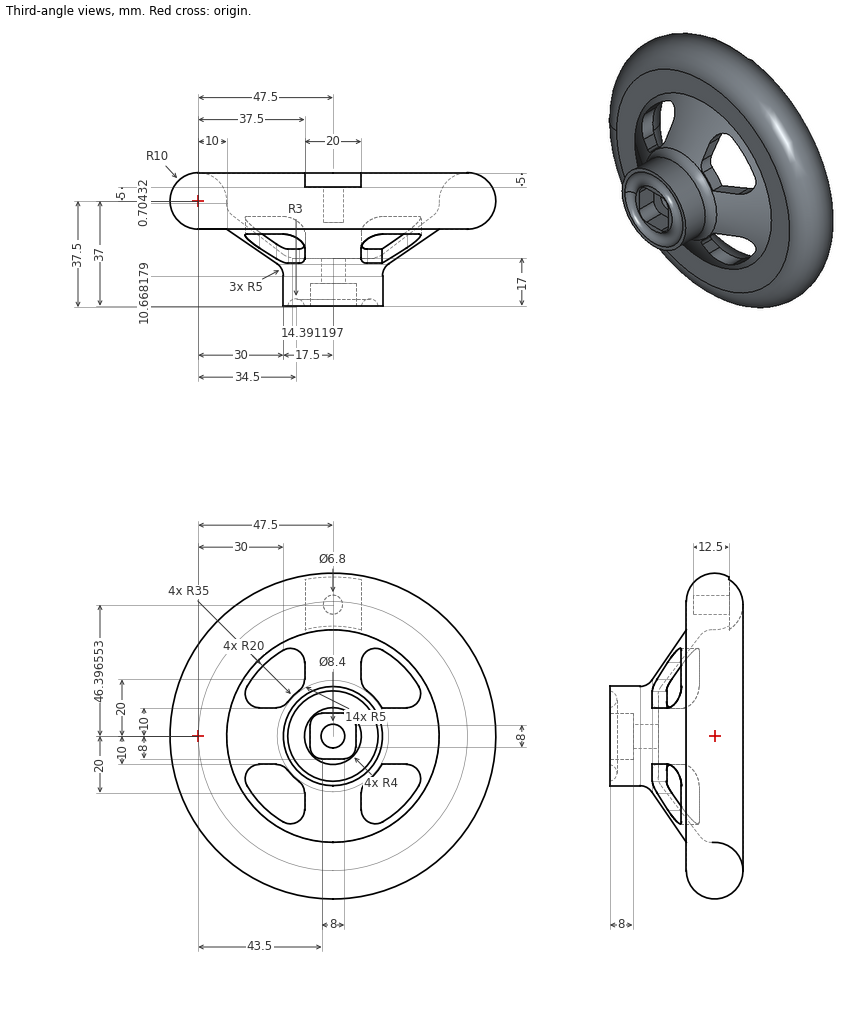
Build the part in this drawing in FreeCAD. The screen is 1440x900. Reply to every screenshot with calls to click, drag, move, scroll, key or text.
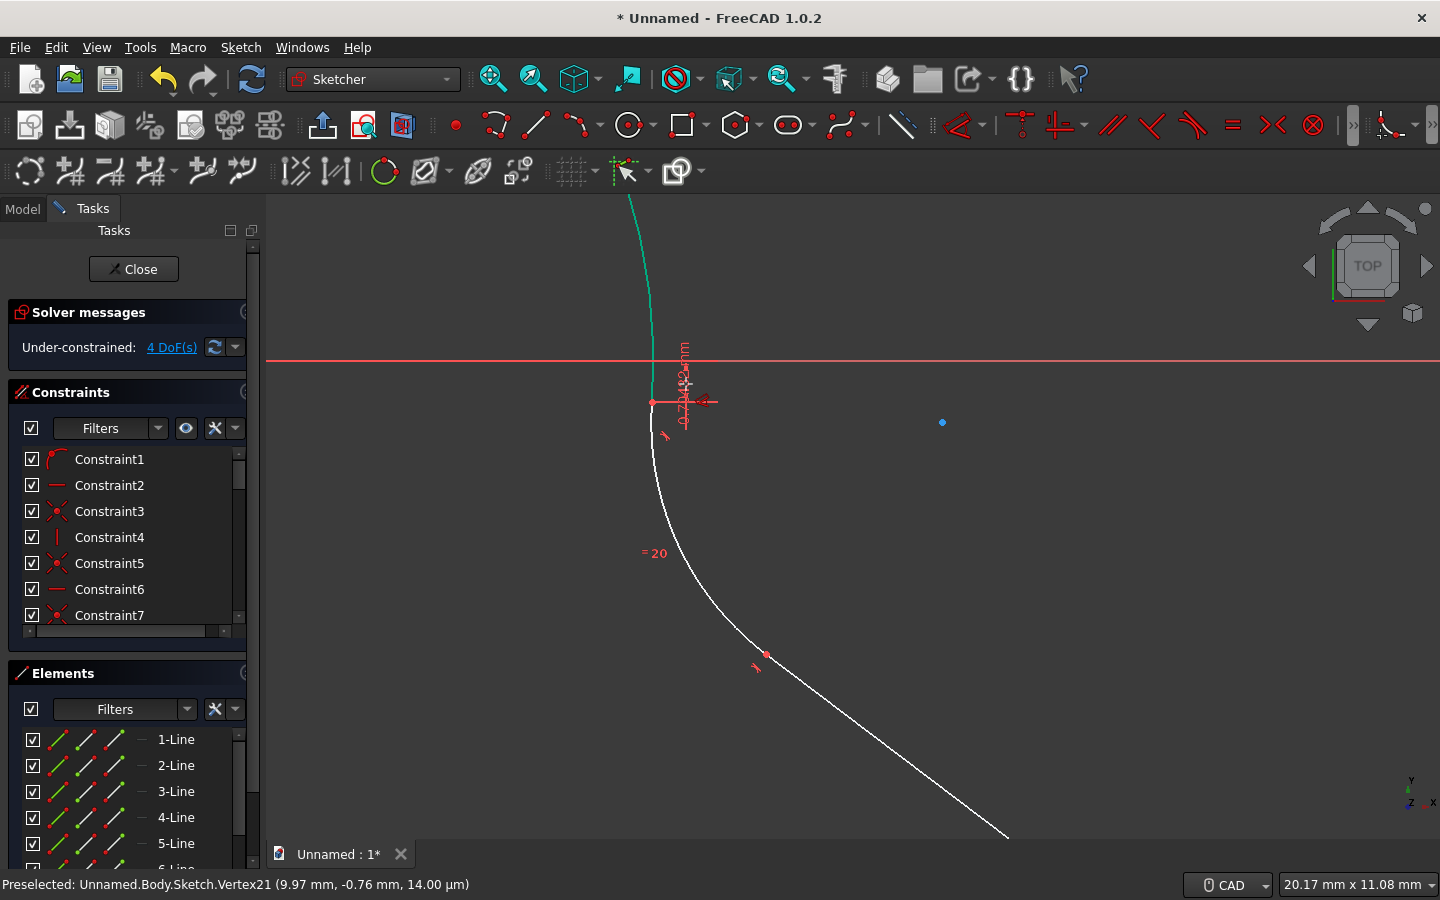
scroll(726, 492, down, 11)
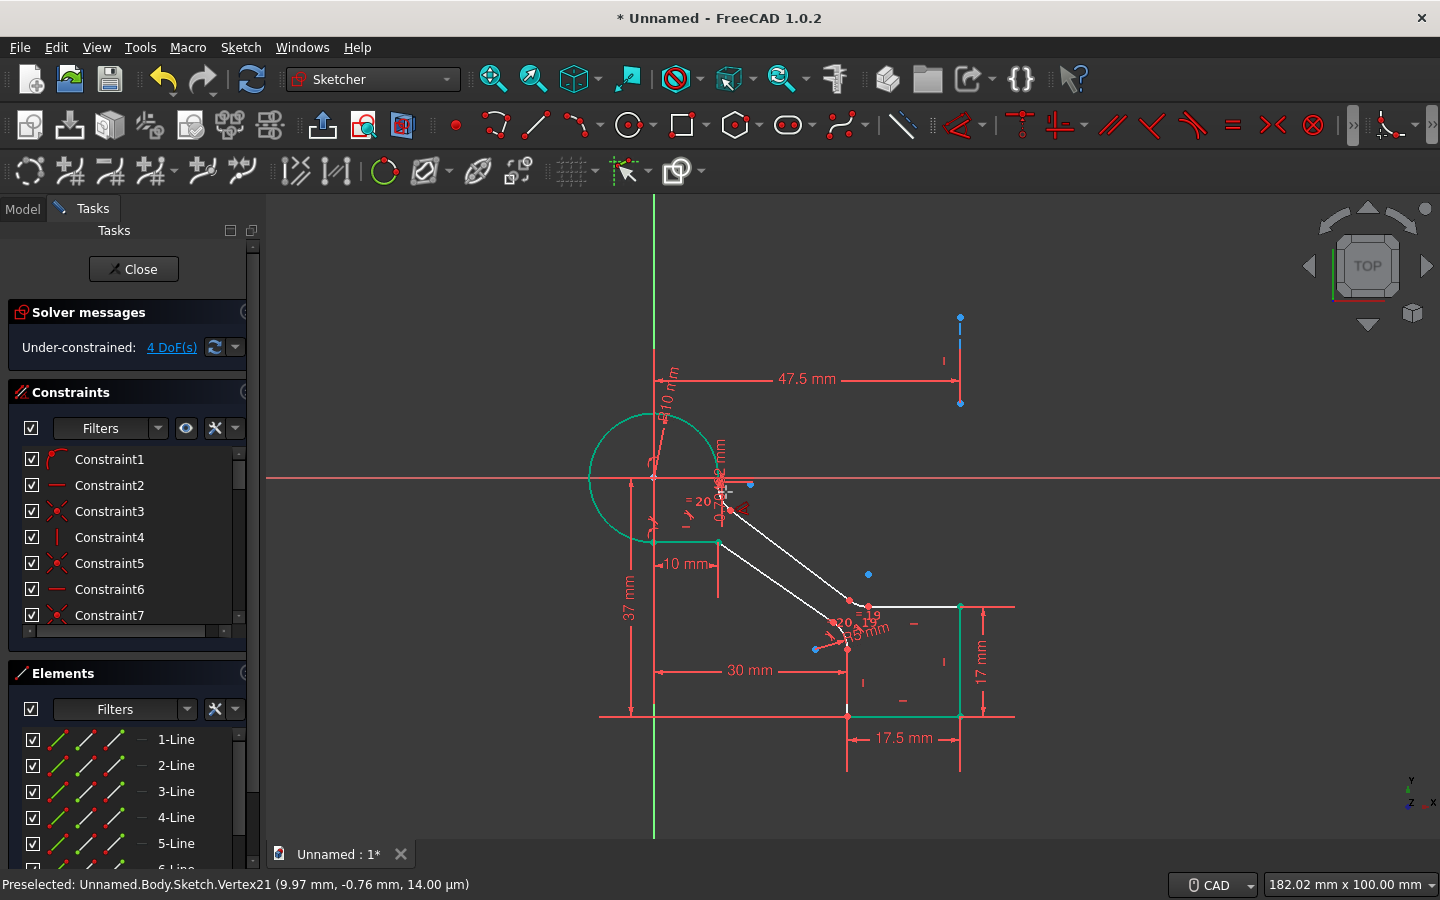
click(847, 669)
click(881, 683)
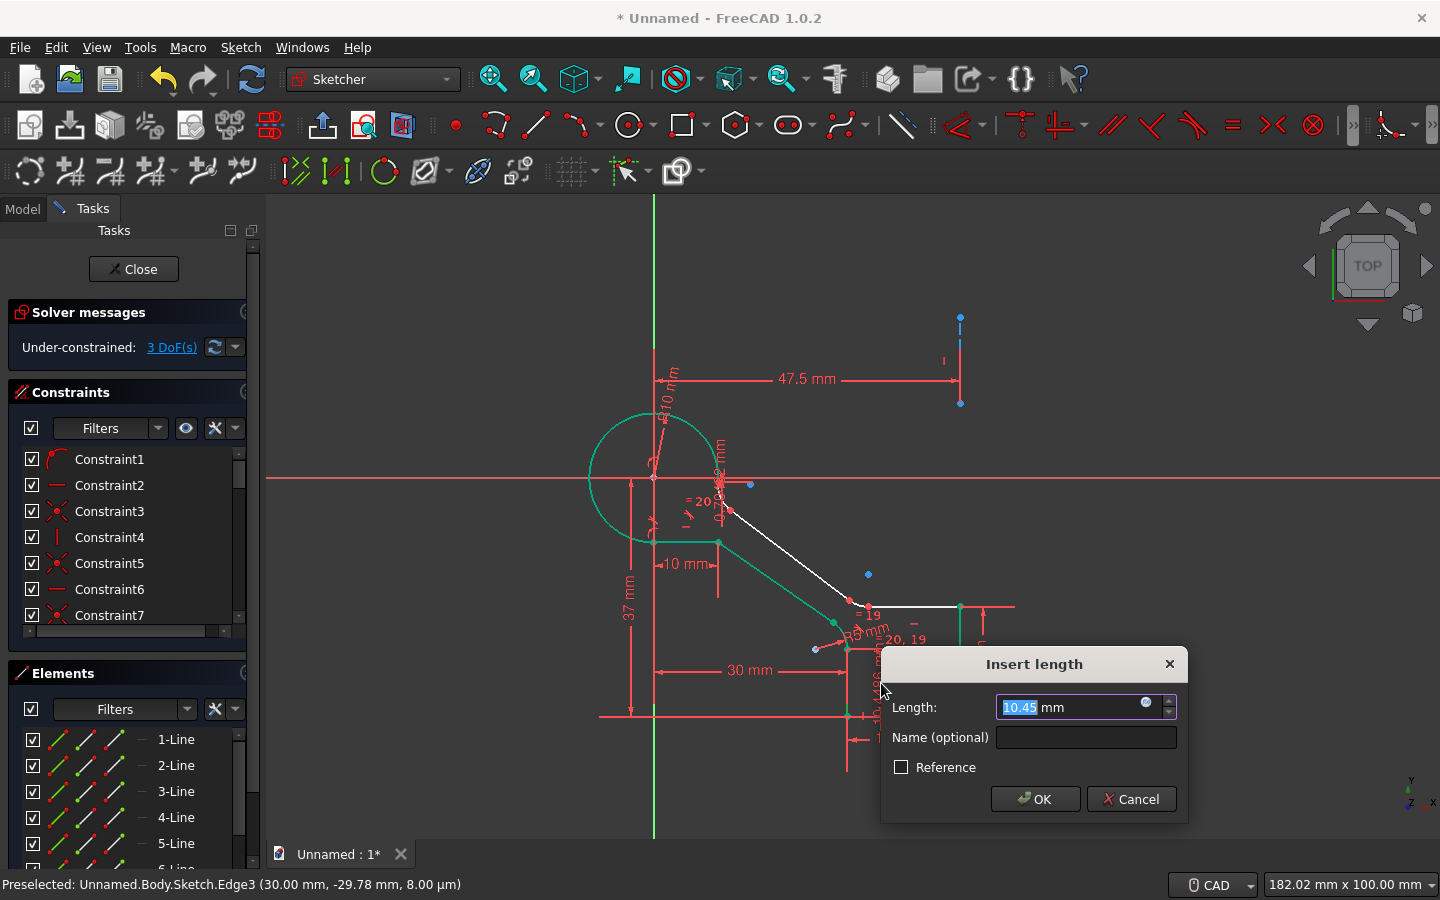
text(10.668179)
key(Return)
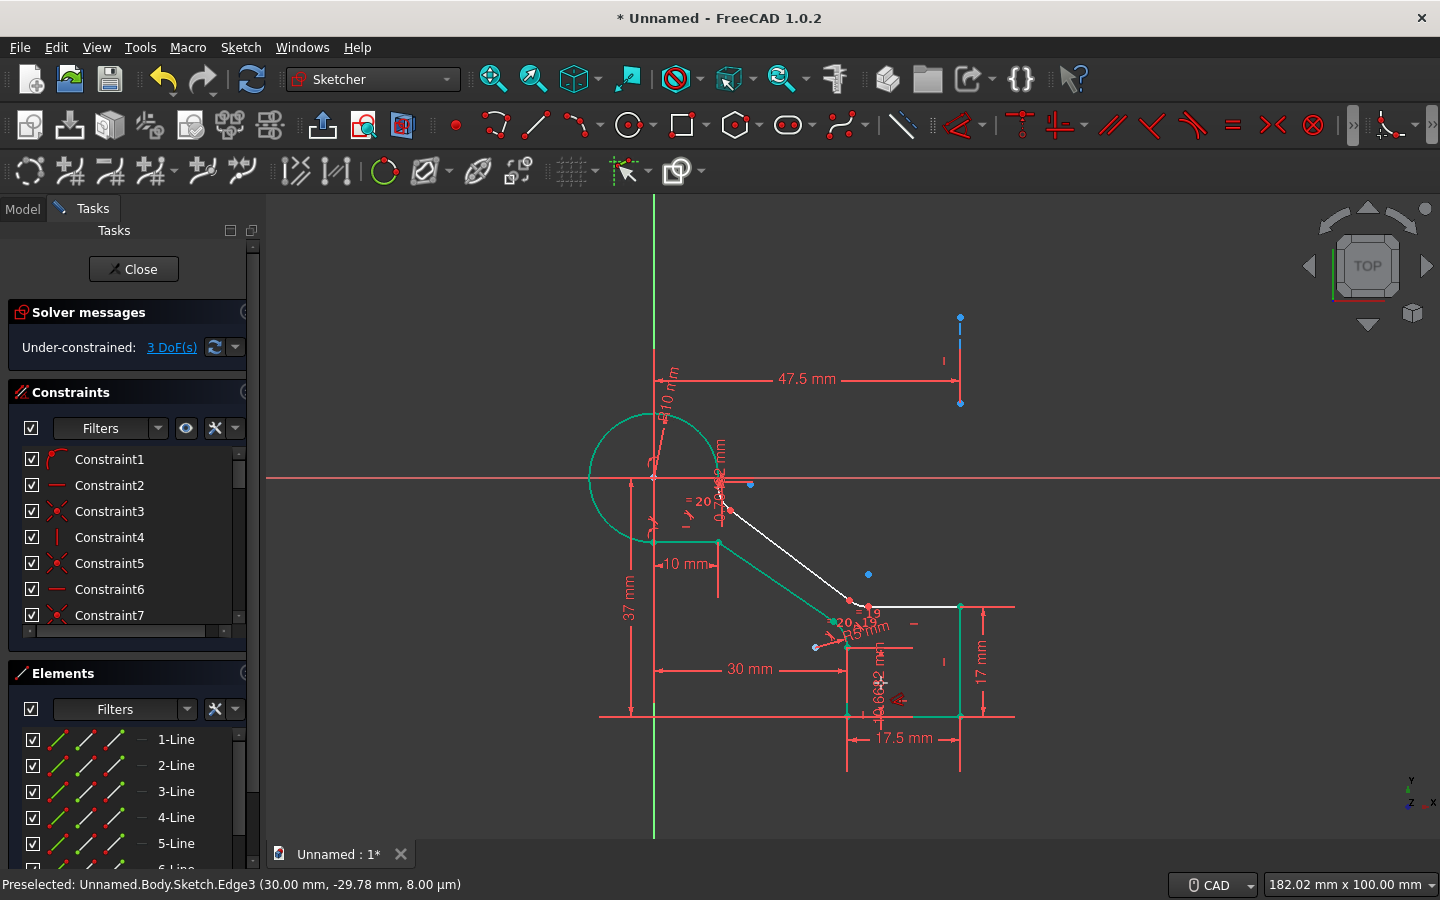
click(933, 607)
click(915, 573)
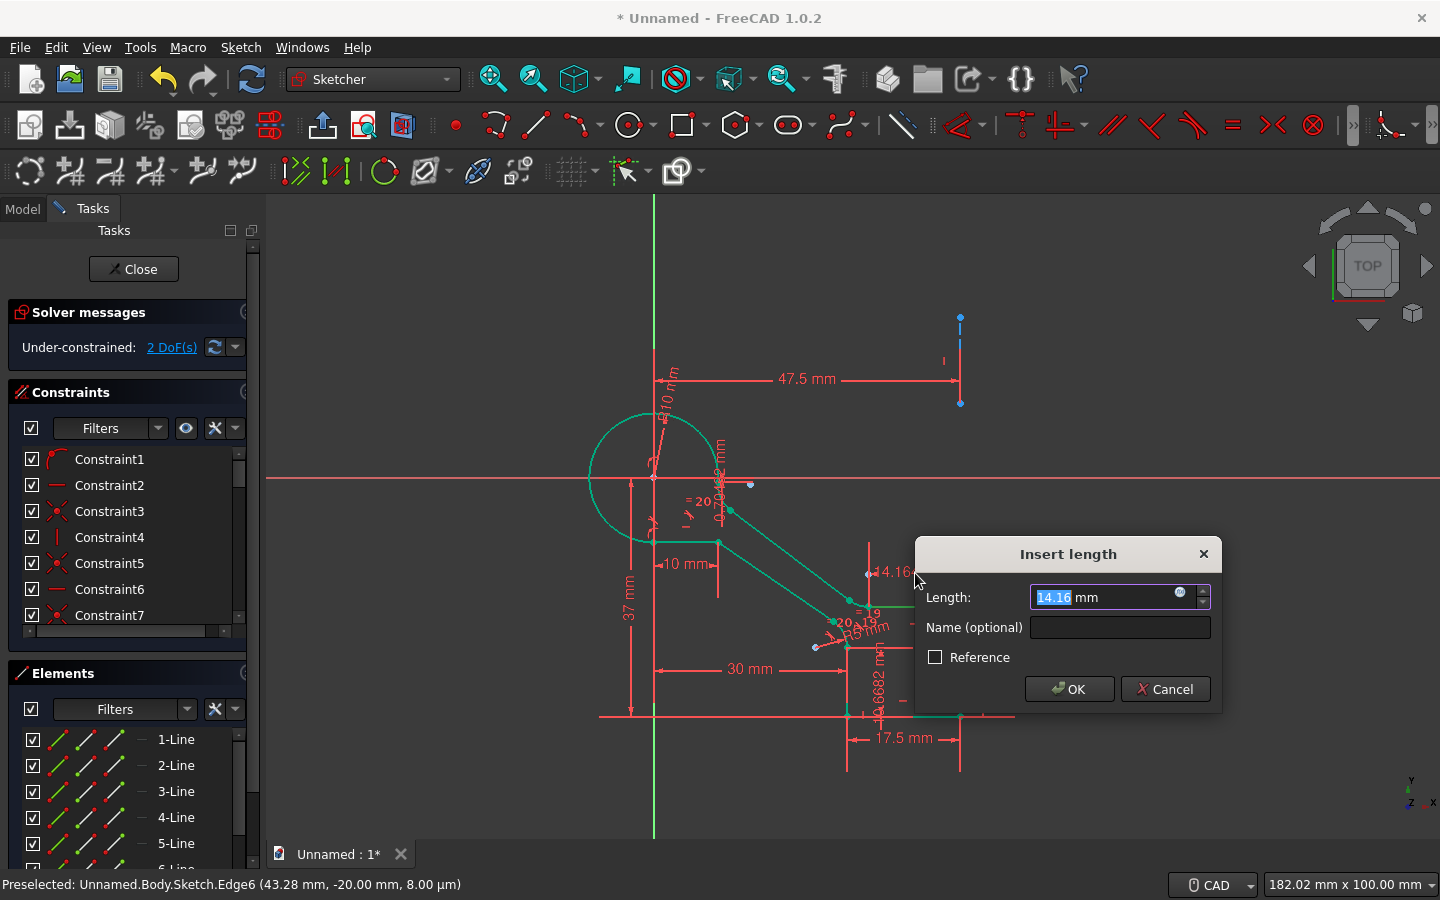
text(14.391197)
key(Return)
key(Escape)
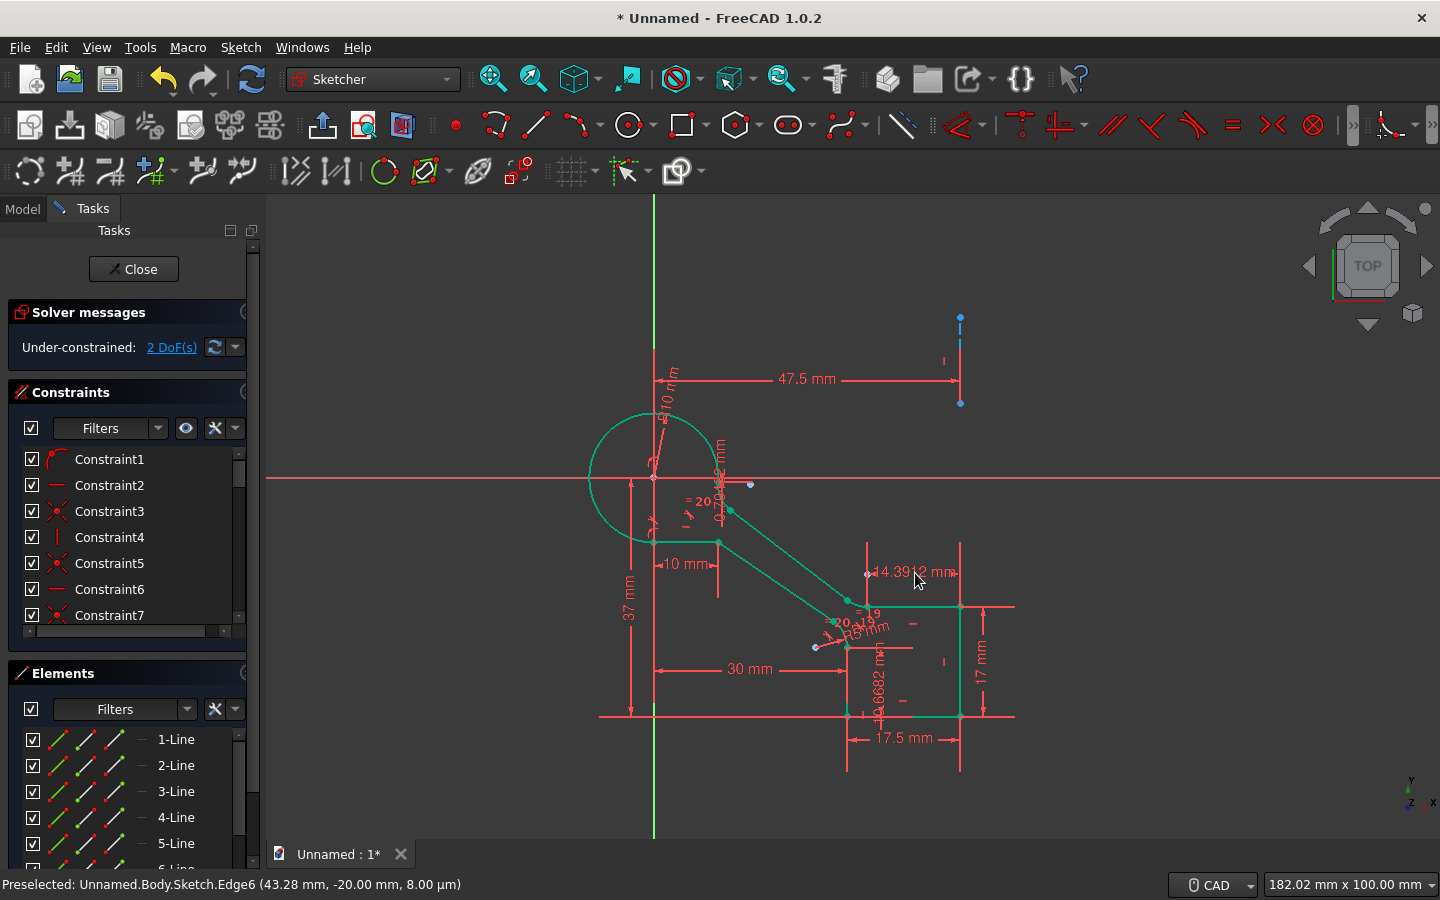
click(134, 269)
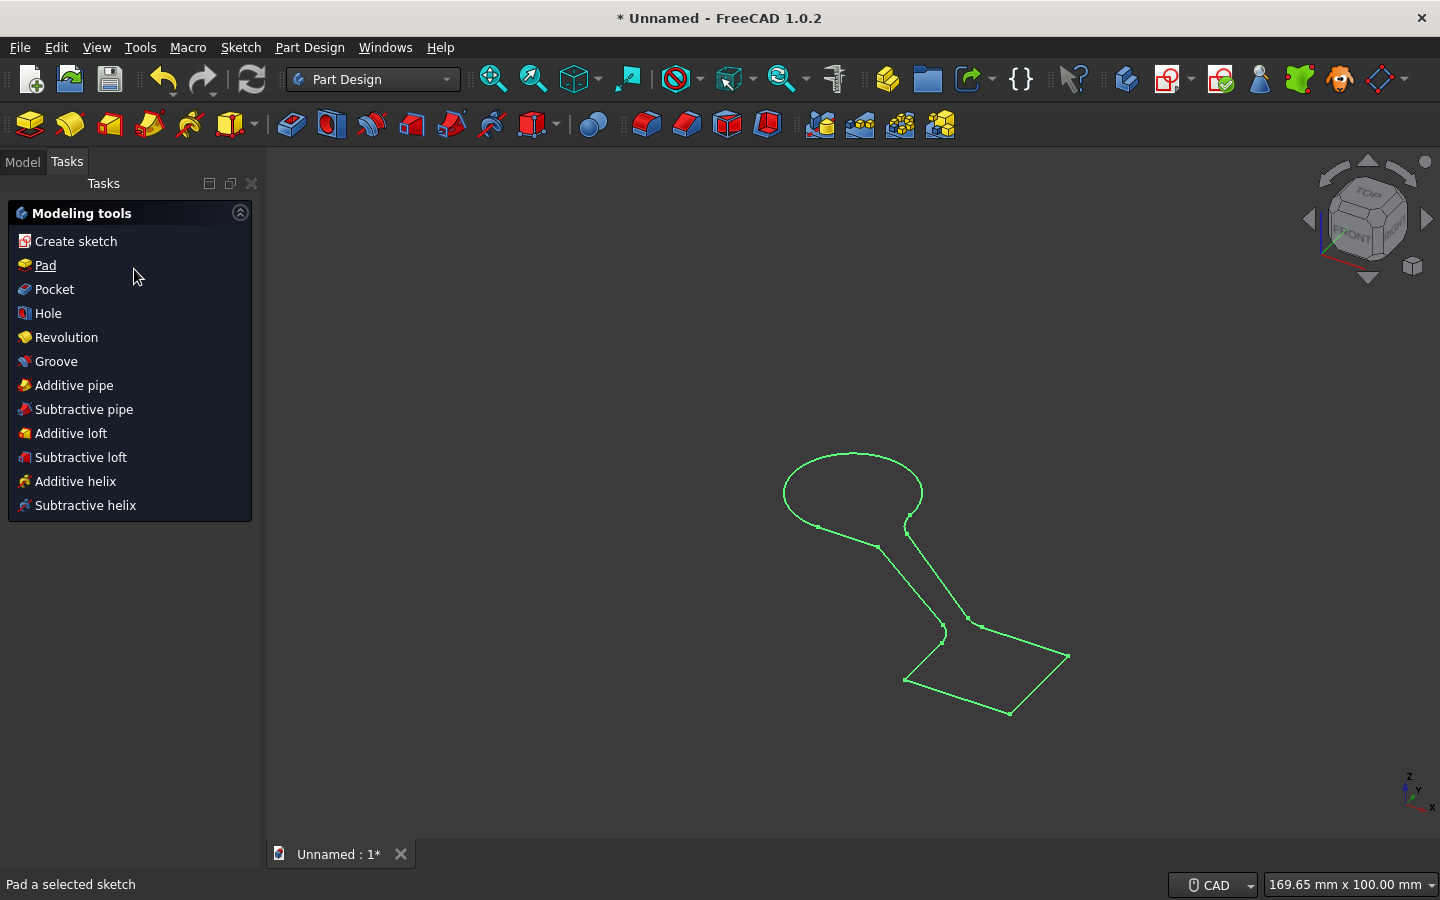
click(70, 124)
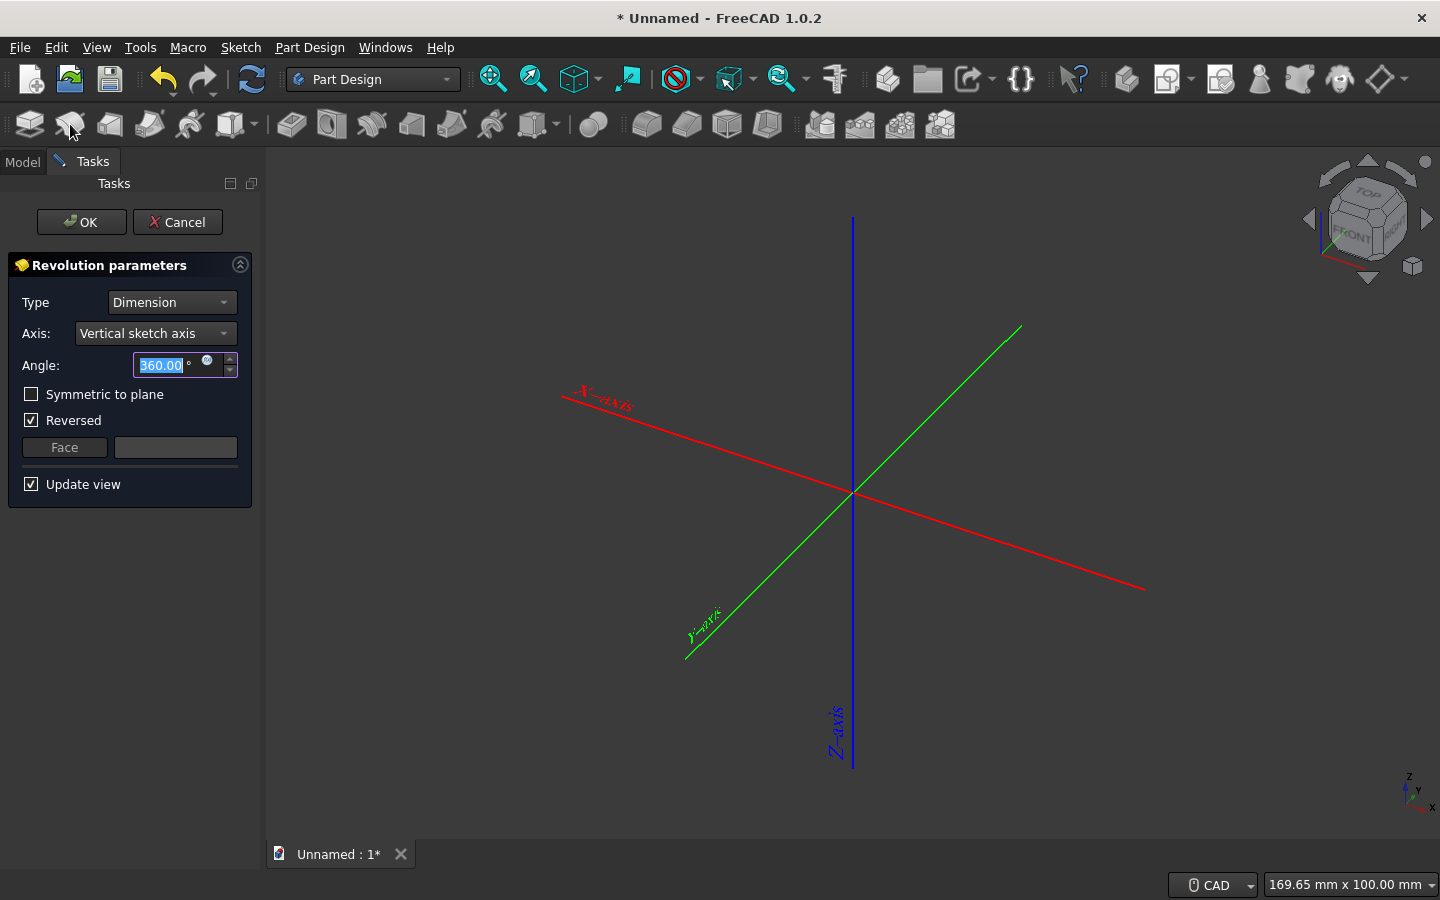
click(156, 334)